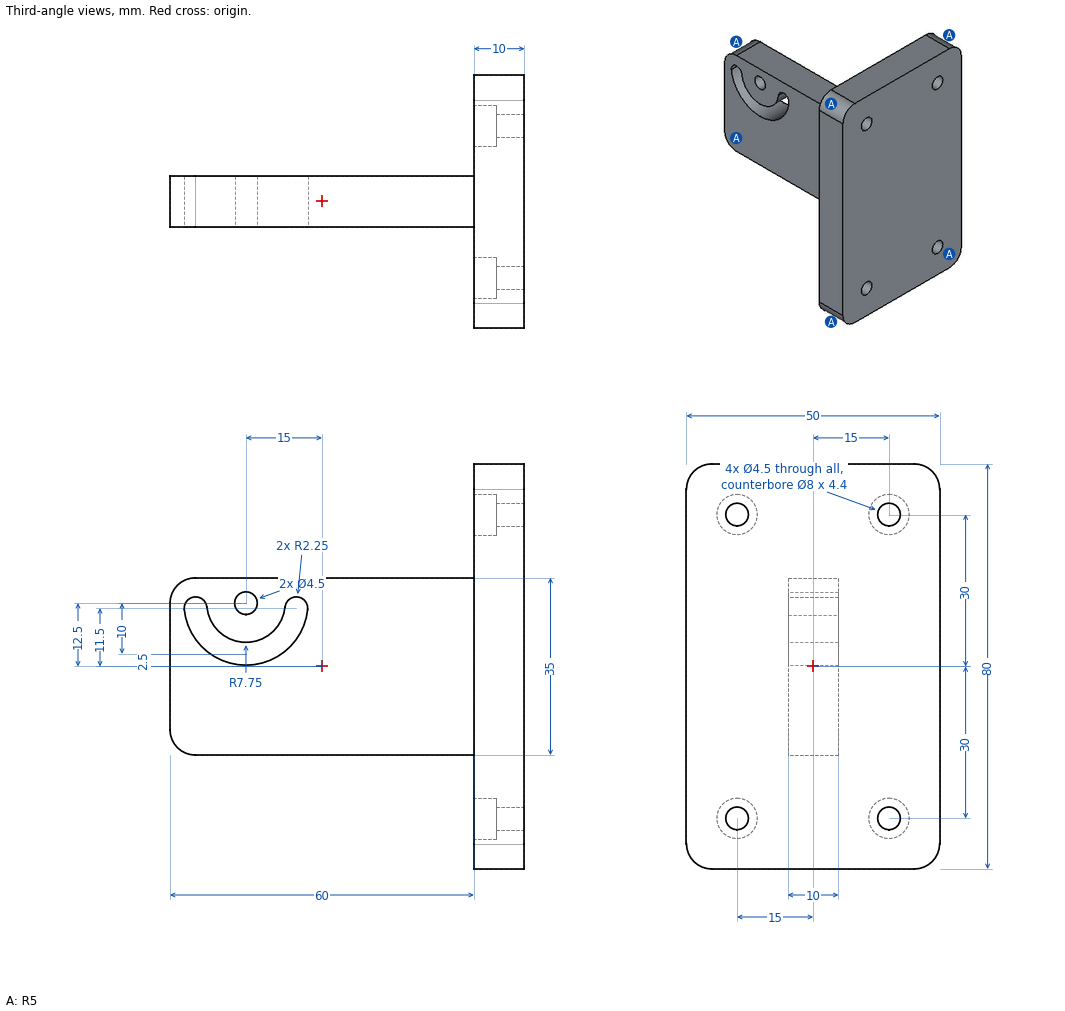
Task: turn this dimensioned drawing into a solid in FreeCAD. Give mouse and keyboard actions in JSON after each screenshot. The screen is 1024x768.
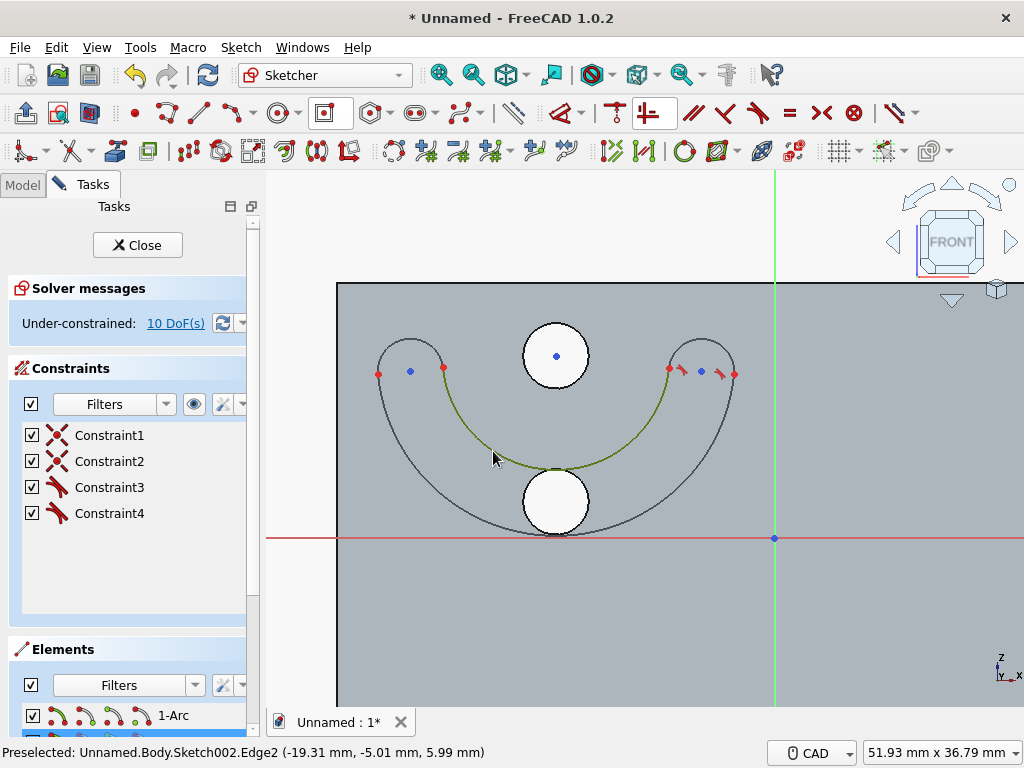
{"action": "left_click", "coordinate": [427, 343]}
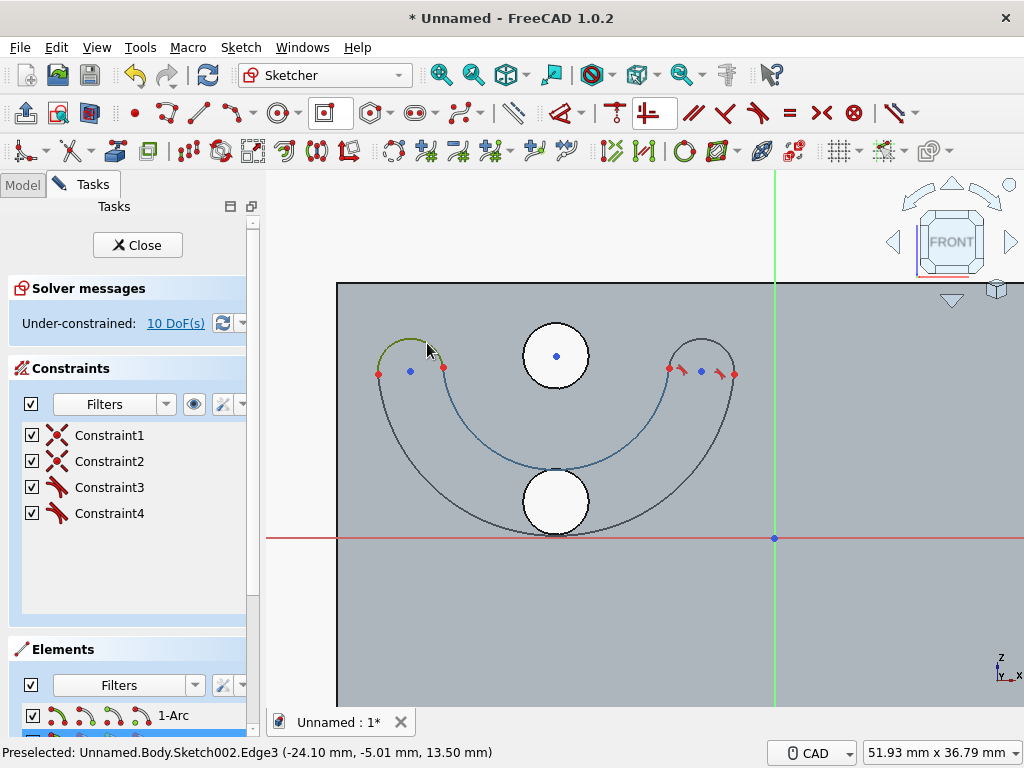
{"action": "left_click", "coordinate": [758, 114]}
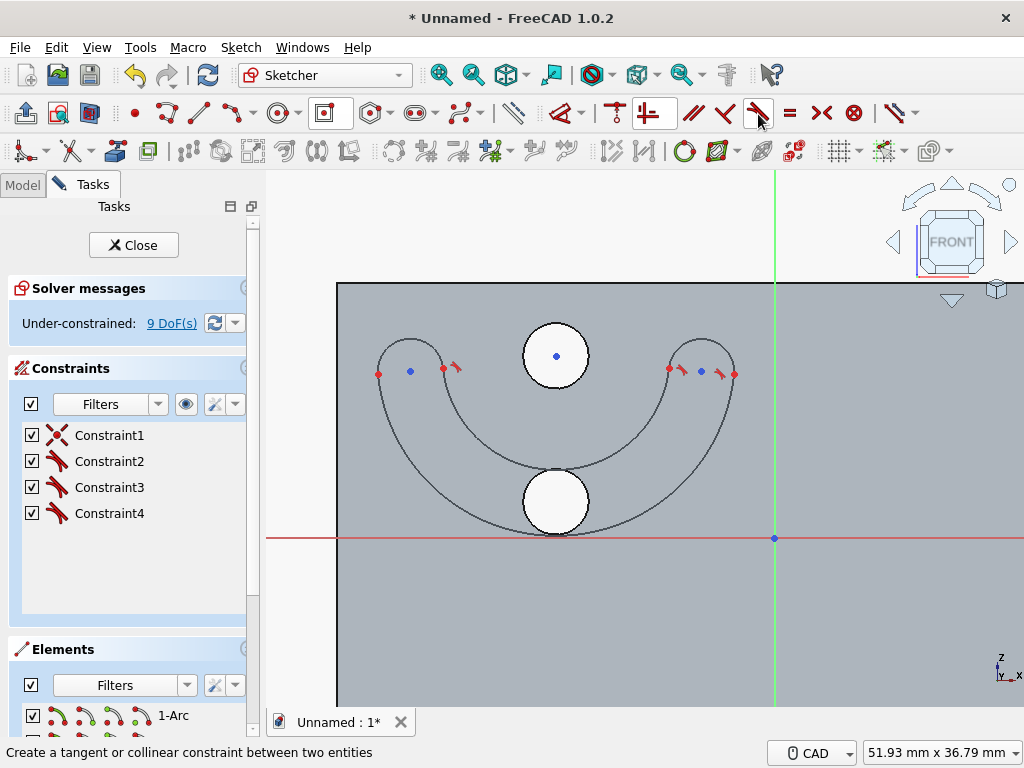
{"action": "left_click", "coordinate": [427, 343]}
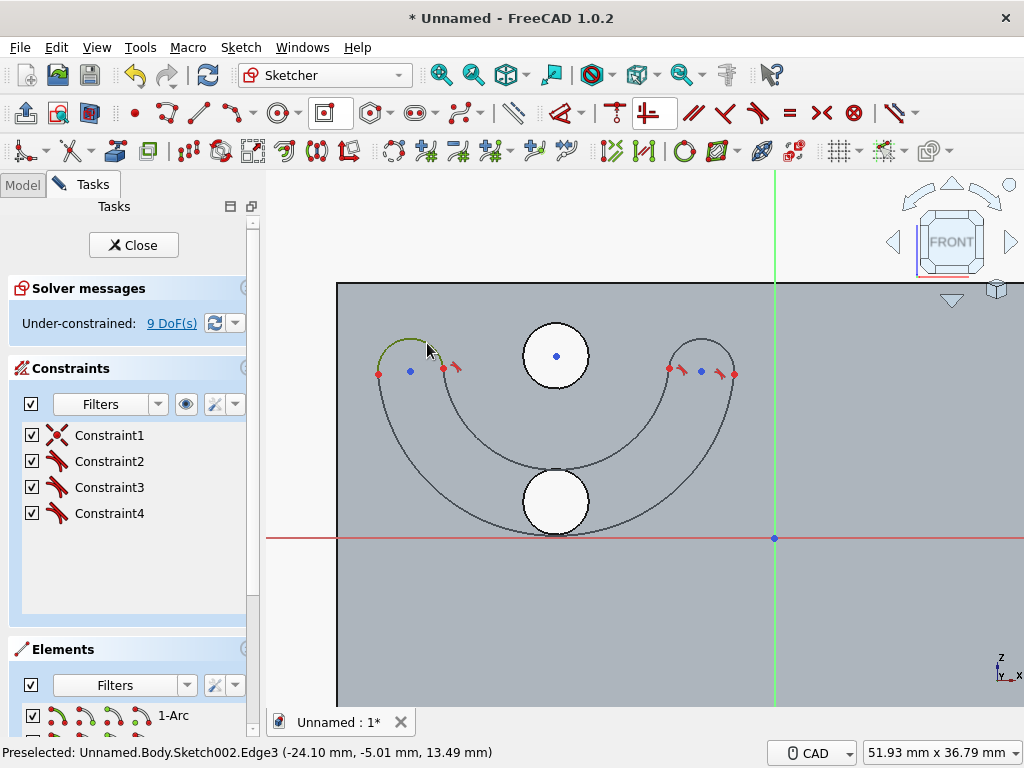
{"action": "left_click", "coordinate": [457, 506]}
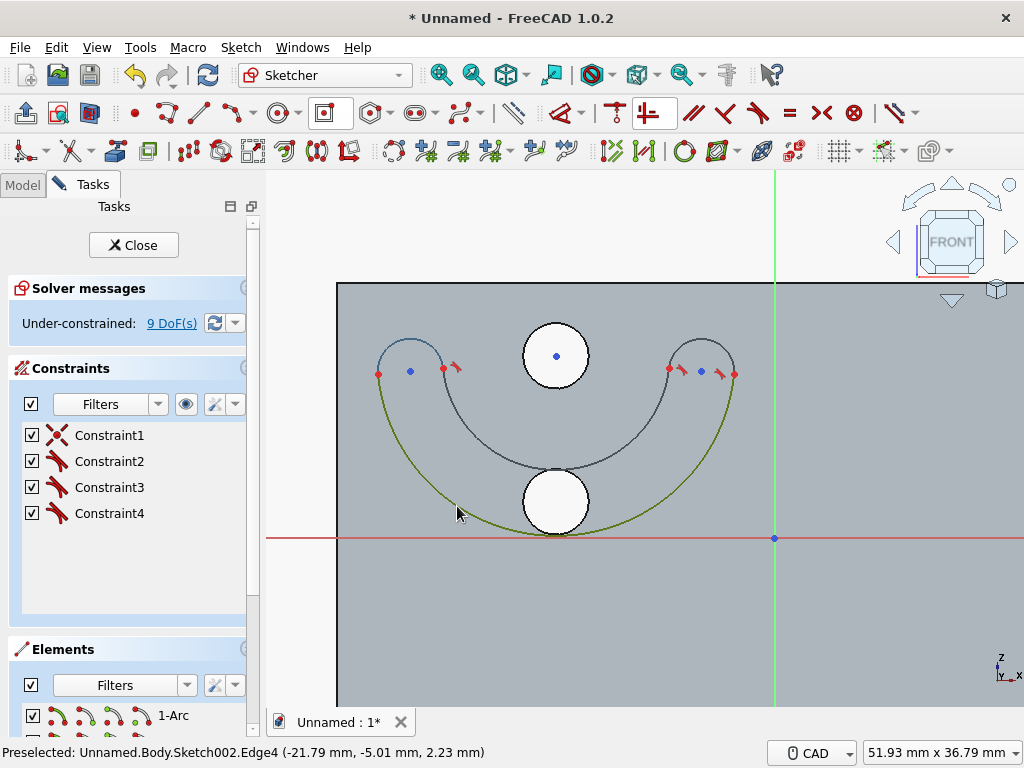
{"action": "left_click", "coordinate": [758, 114]}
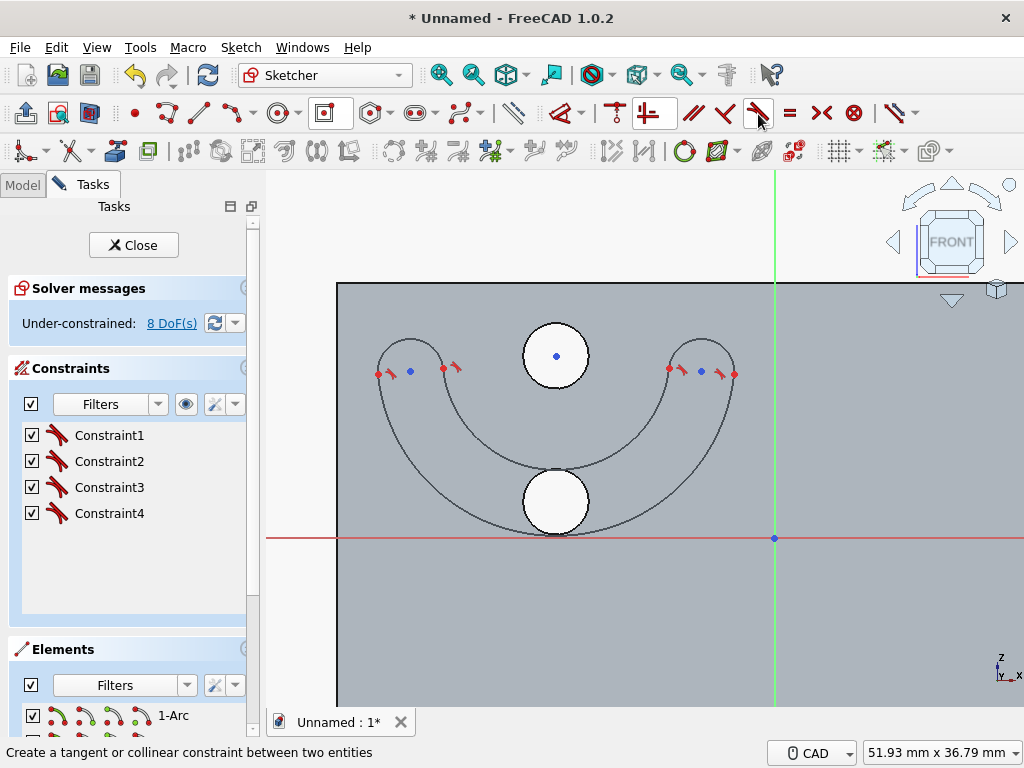
{"action": "left_click", "coordinate": [493, 451]}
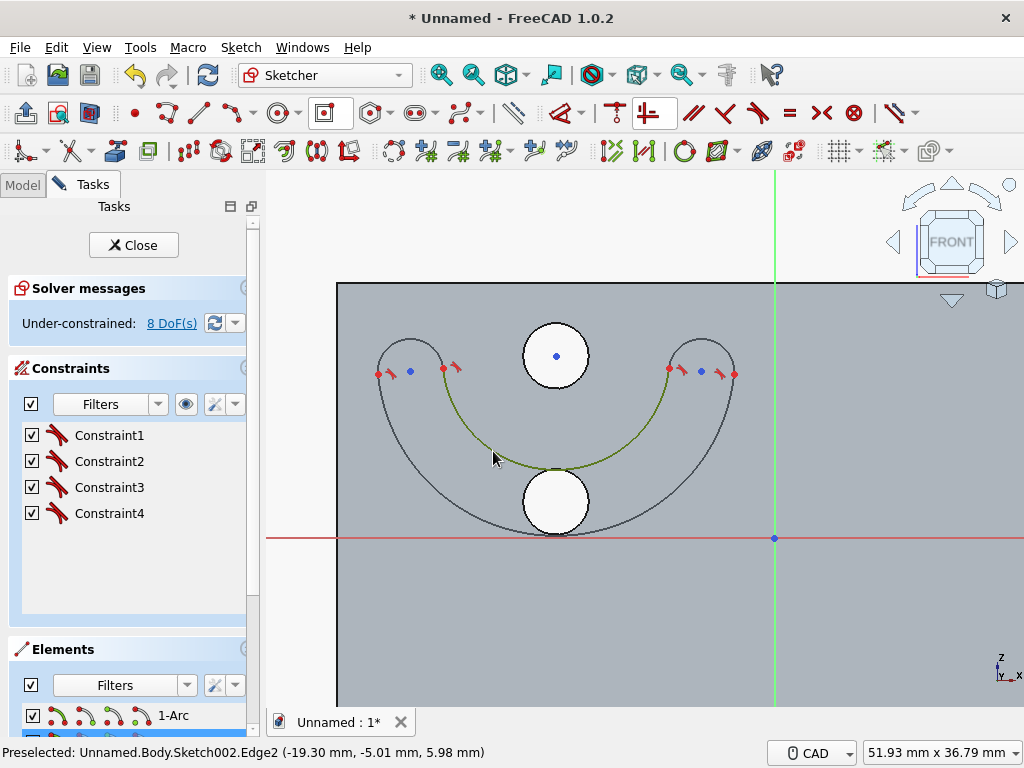
{"action": "left_click", "coordinate": [457, 506]}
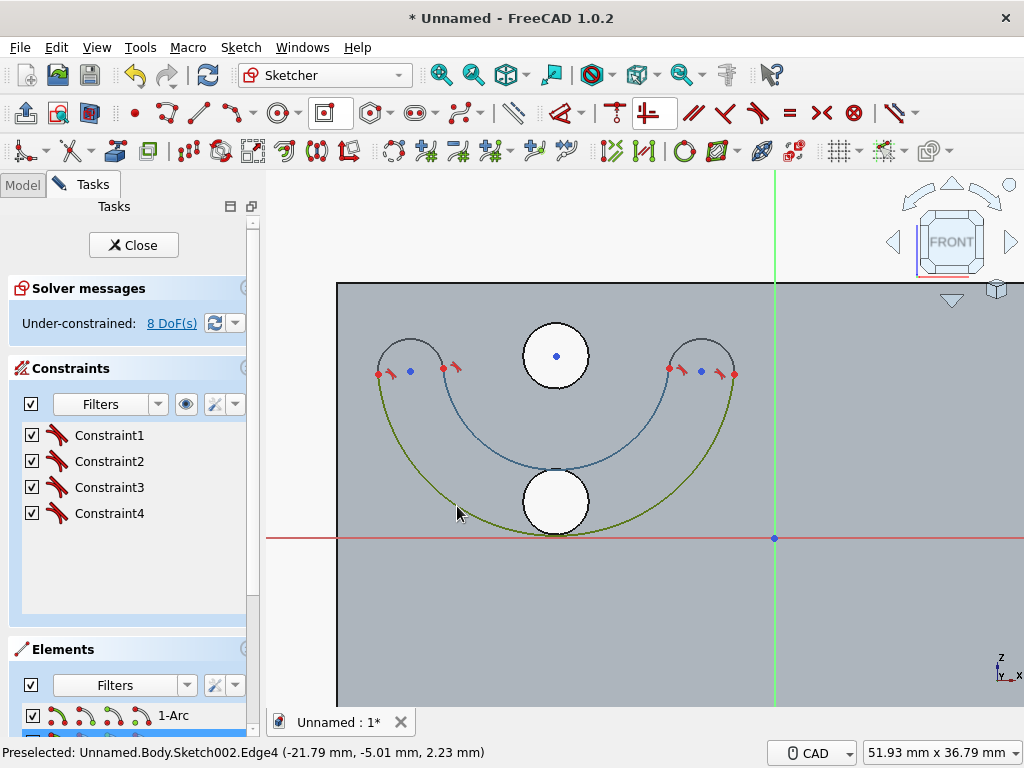
{"action": "left_click", "coordinate": [616, 114]}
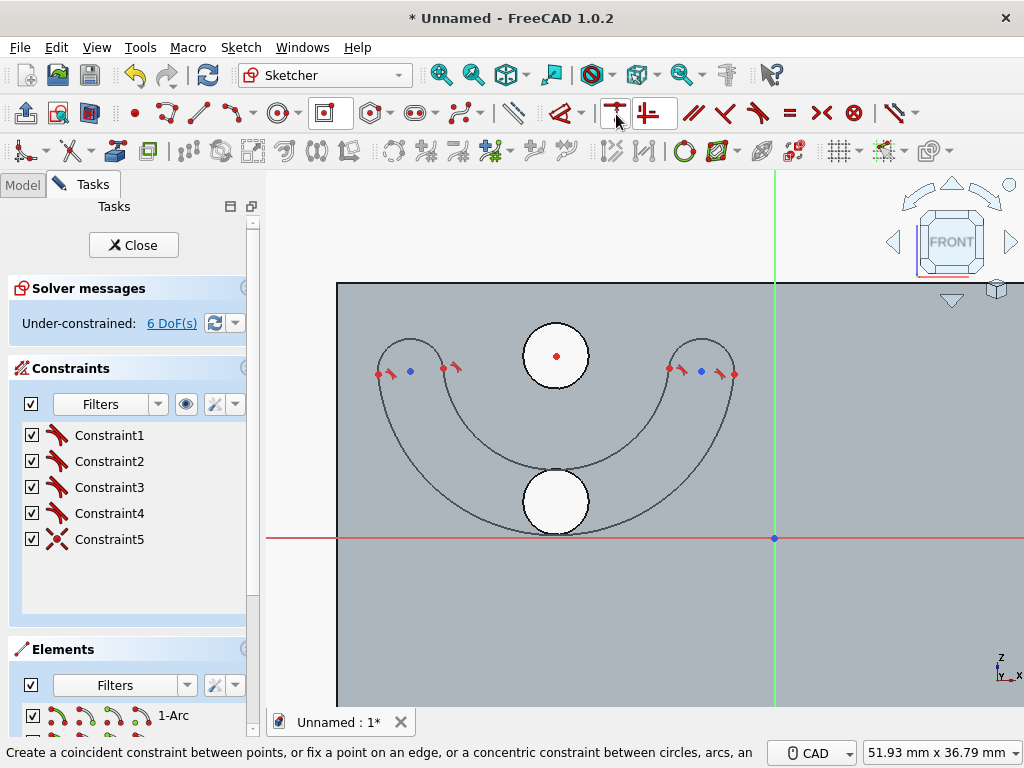
{"action": "left_click", "coordinate": [560, 114]}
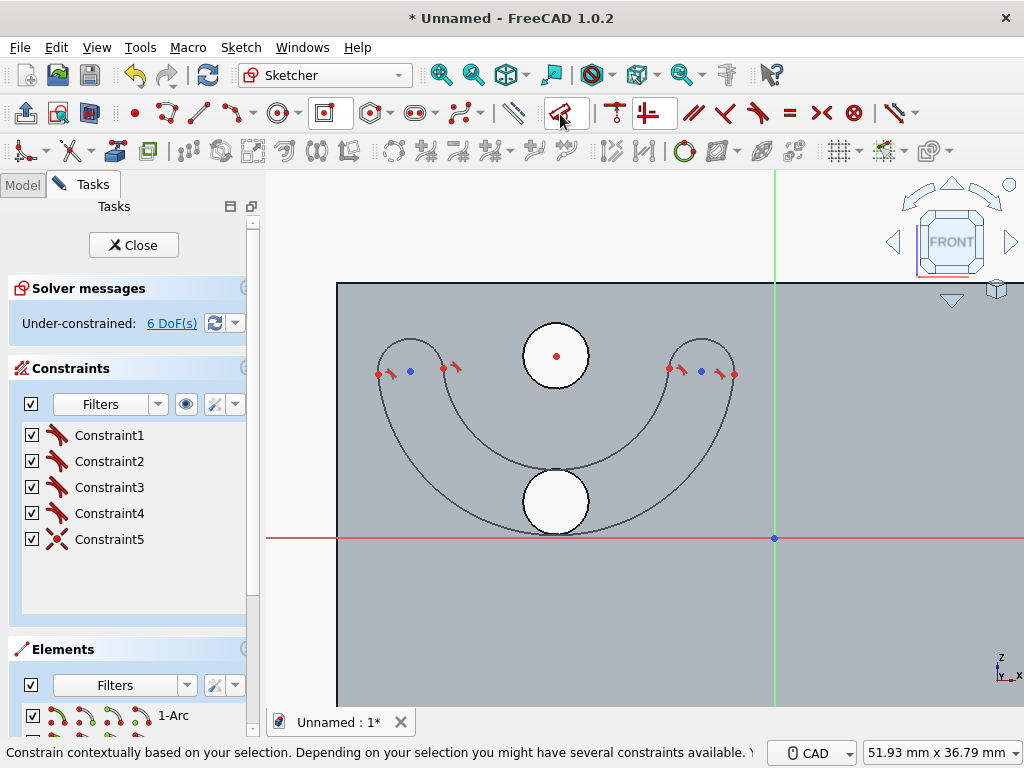
{"action": "left_click", "coordinate": [723, 347]}
{"action": "left_click", "coordinate": [744, 323]}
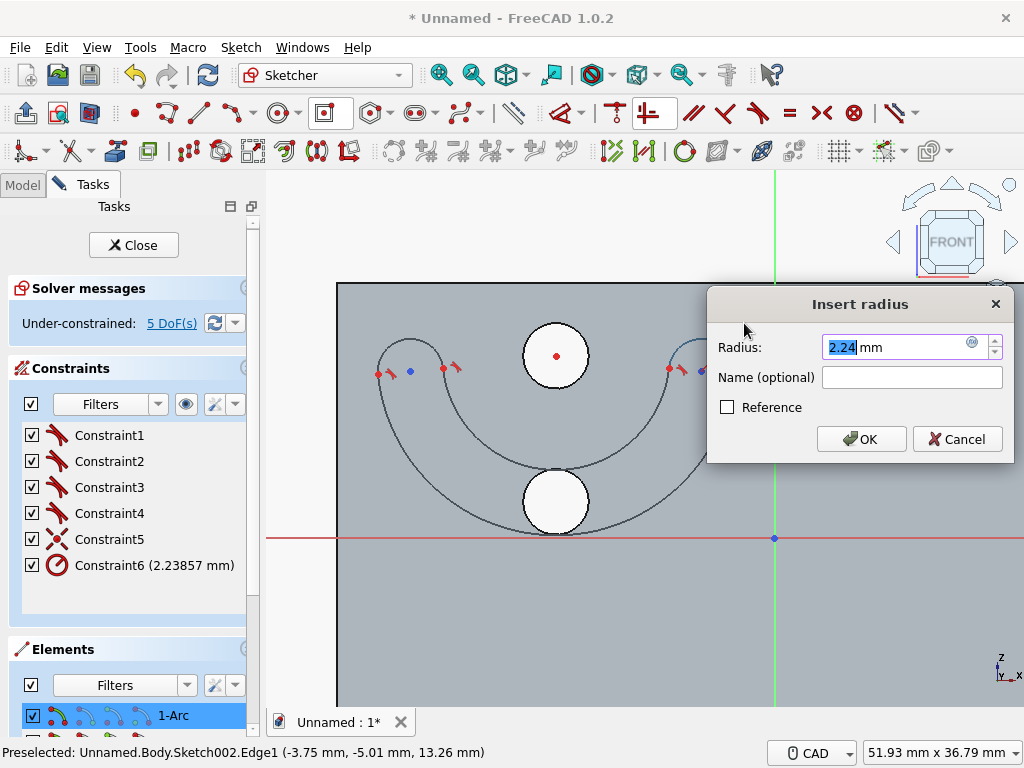
{"action": "type", "text": "2.25"}
{"action": "key", "text": "Return"}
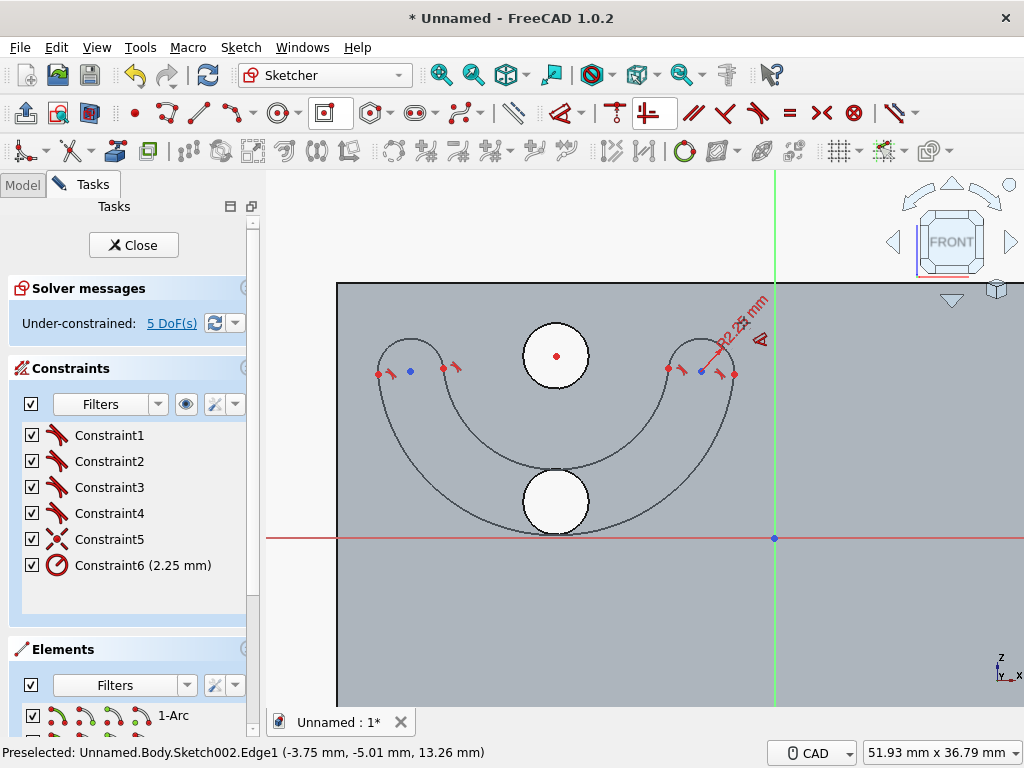
{"action": "left_click", "coordinate": [493, 451]}
{"action": "left_click", "coordinate": [475, 478]}